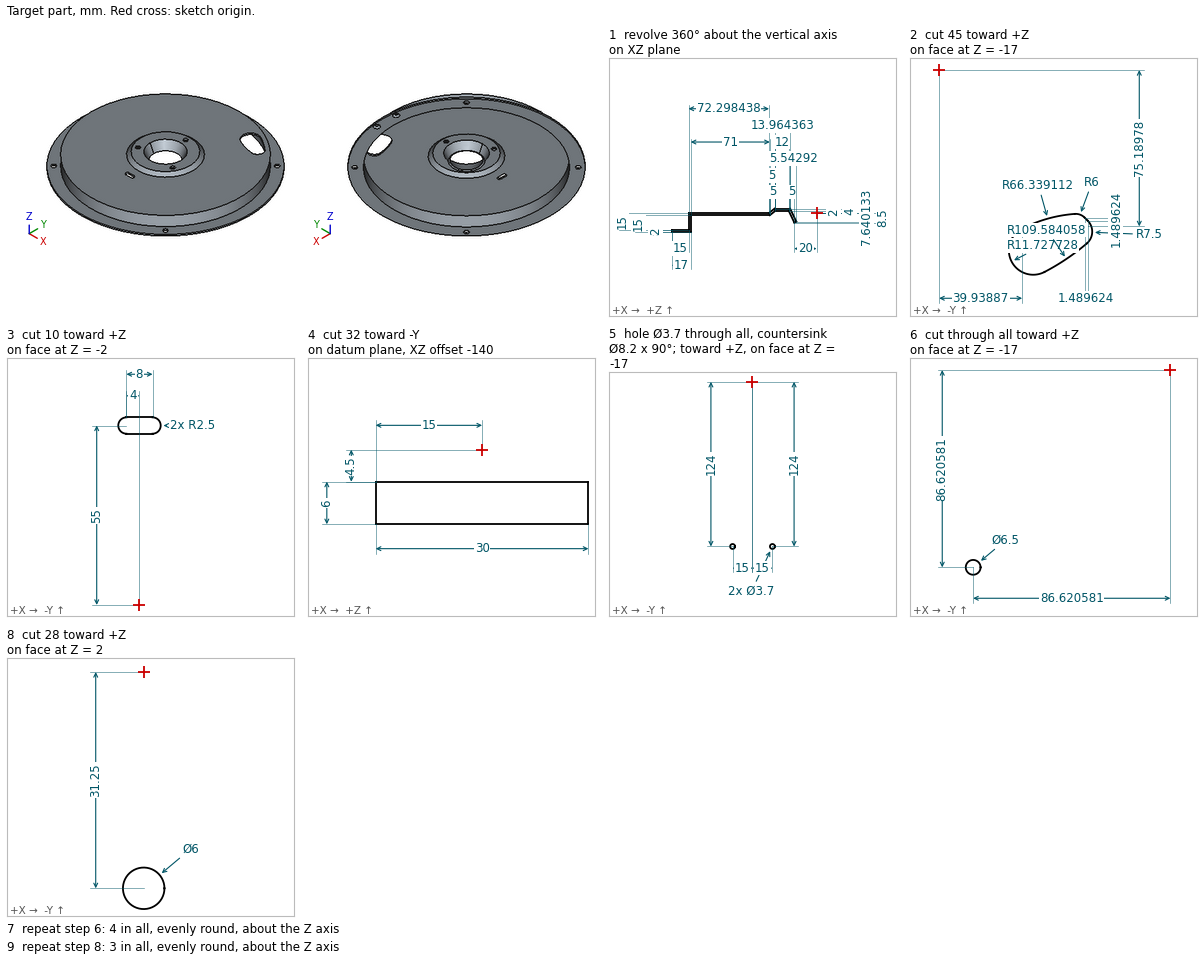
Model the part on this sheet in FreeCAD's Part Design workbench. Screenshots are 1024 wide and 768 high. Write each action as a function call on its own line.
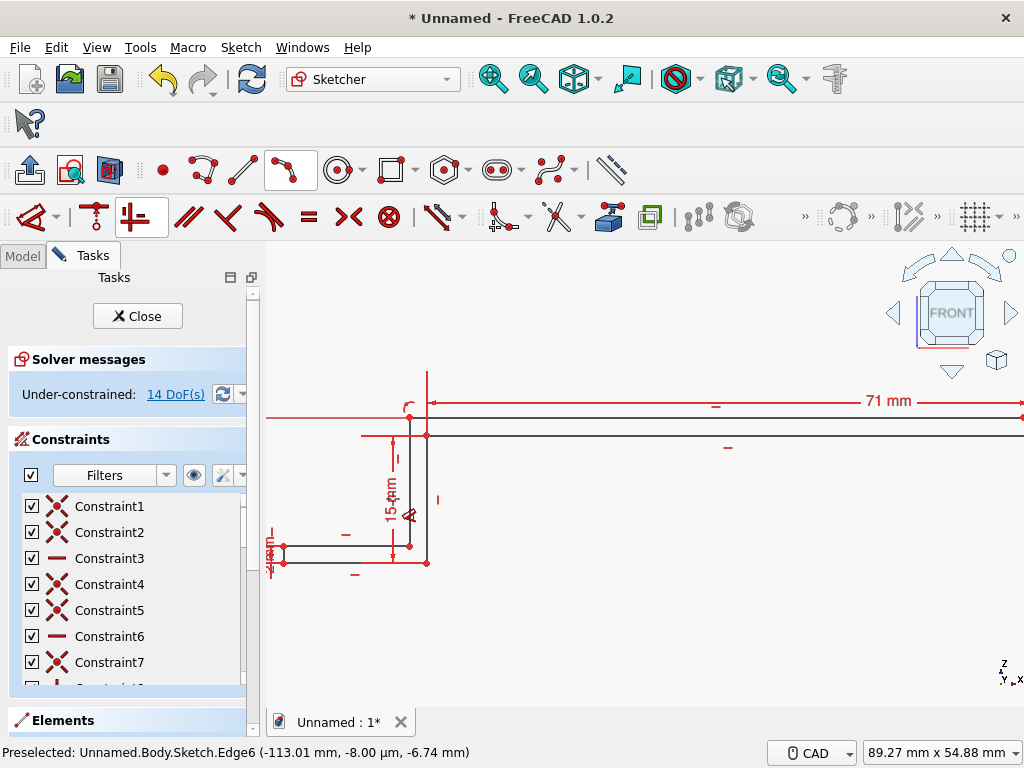
click(384, 563)
click(360, 597)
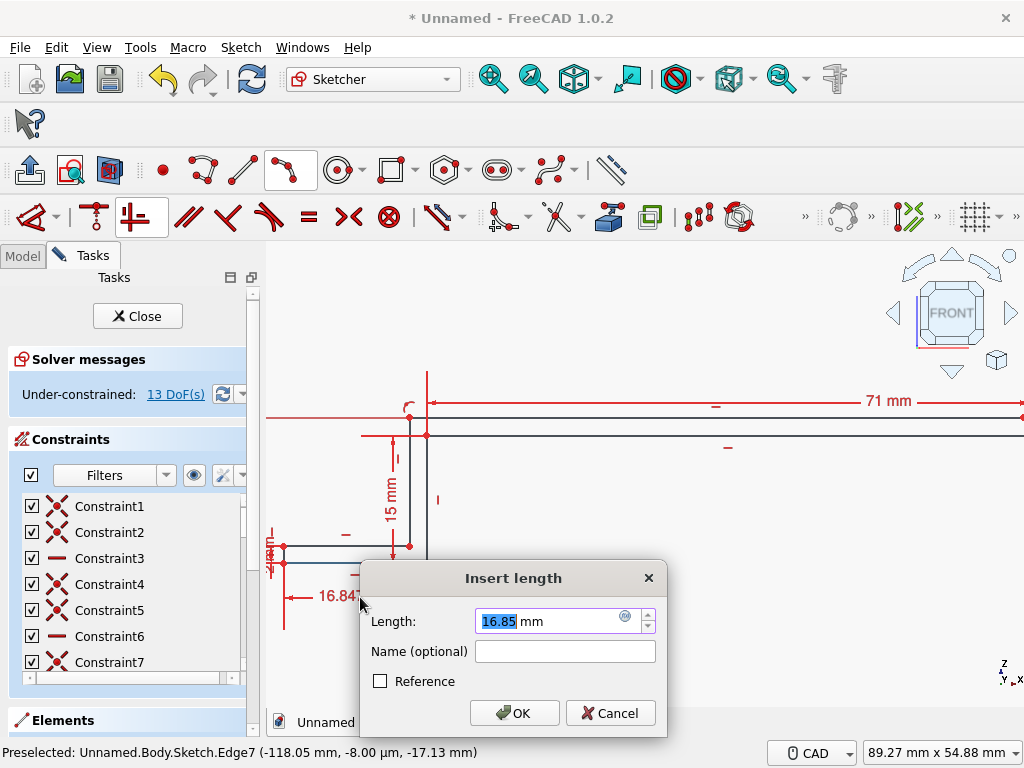
text(17)
key(Return)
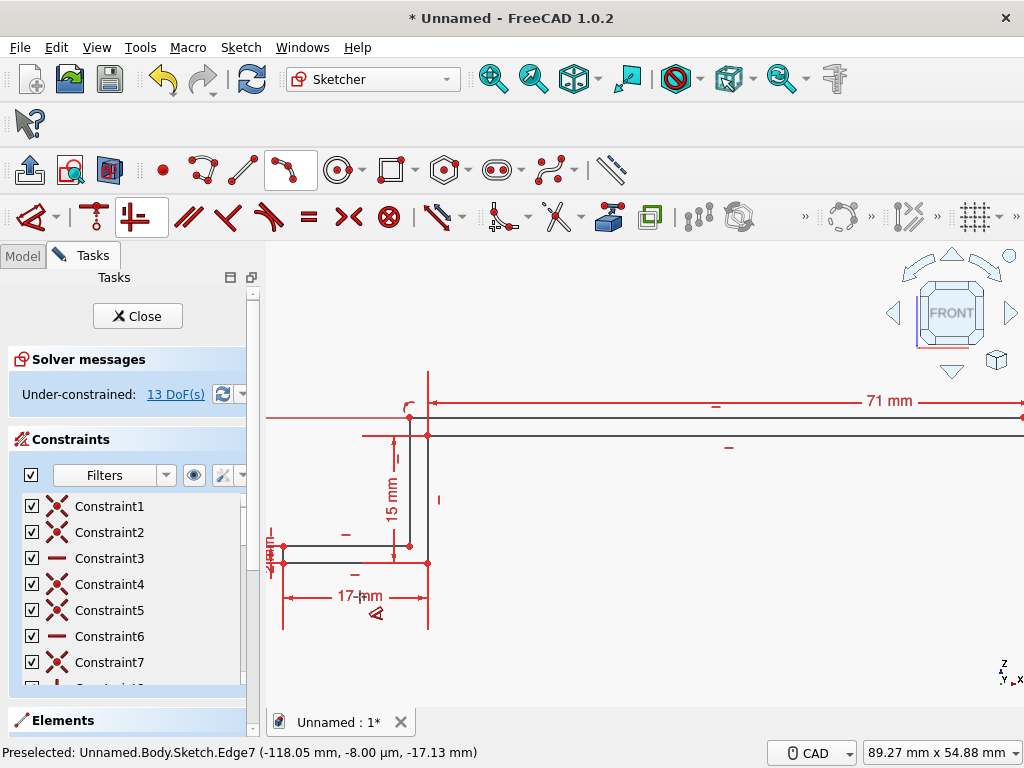
click(321, 546)
click(311, 512)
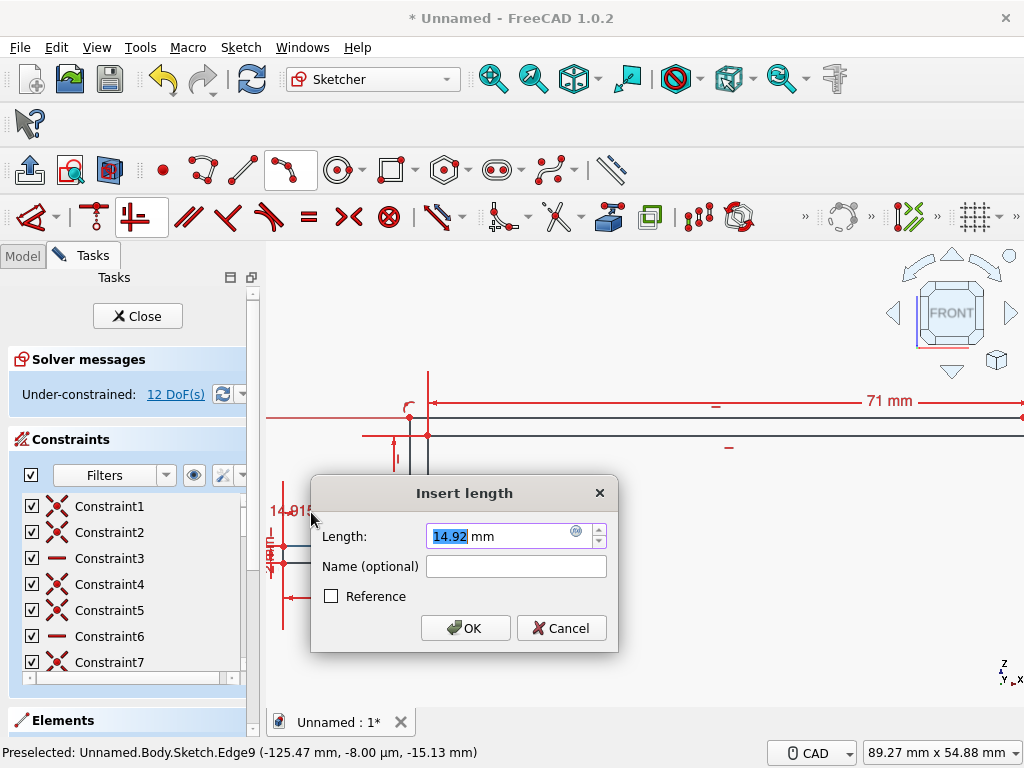
text(15)
key(Return)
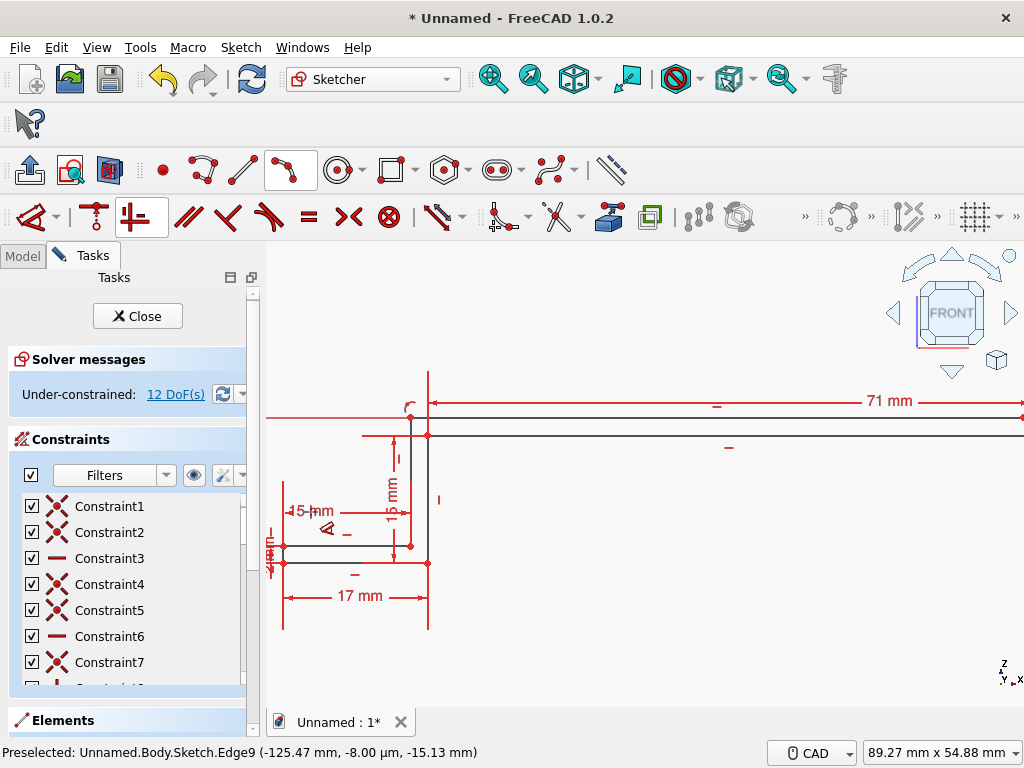
click(411, 508)
click(377, 452)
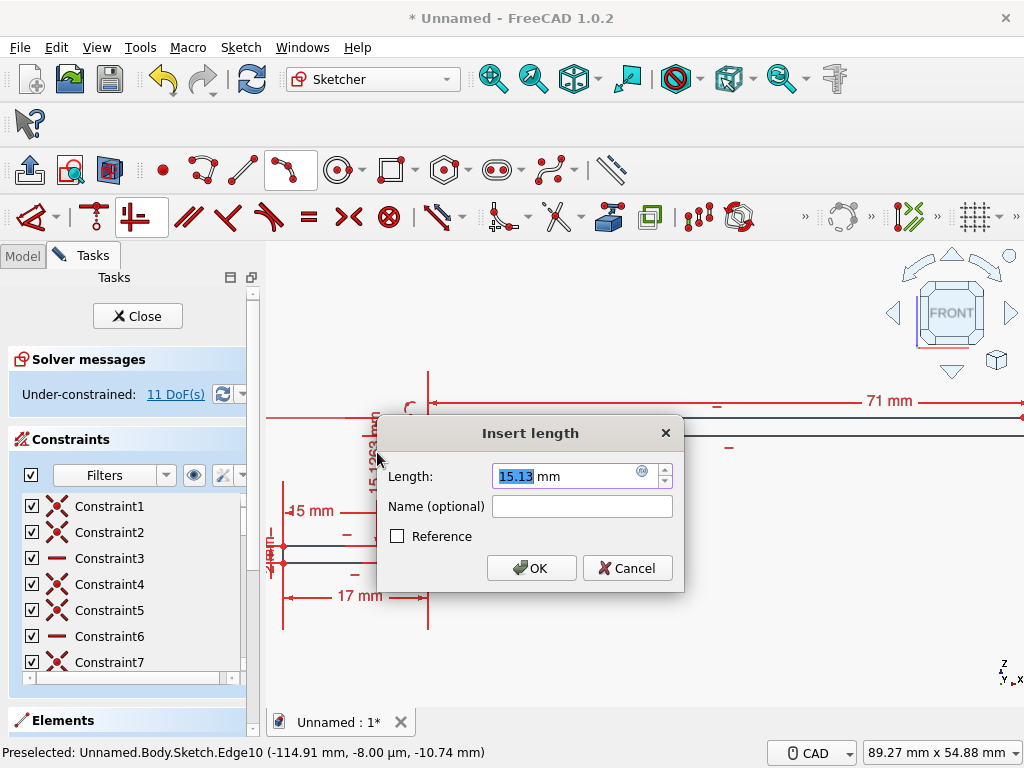
text(15)
key(Return)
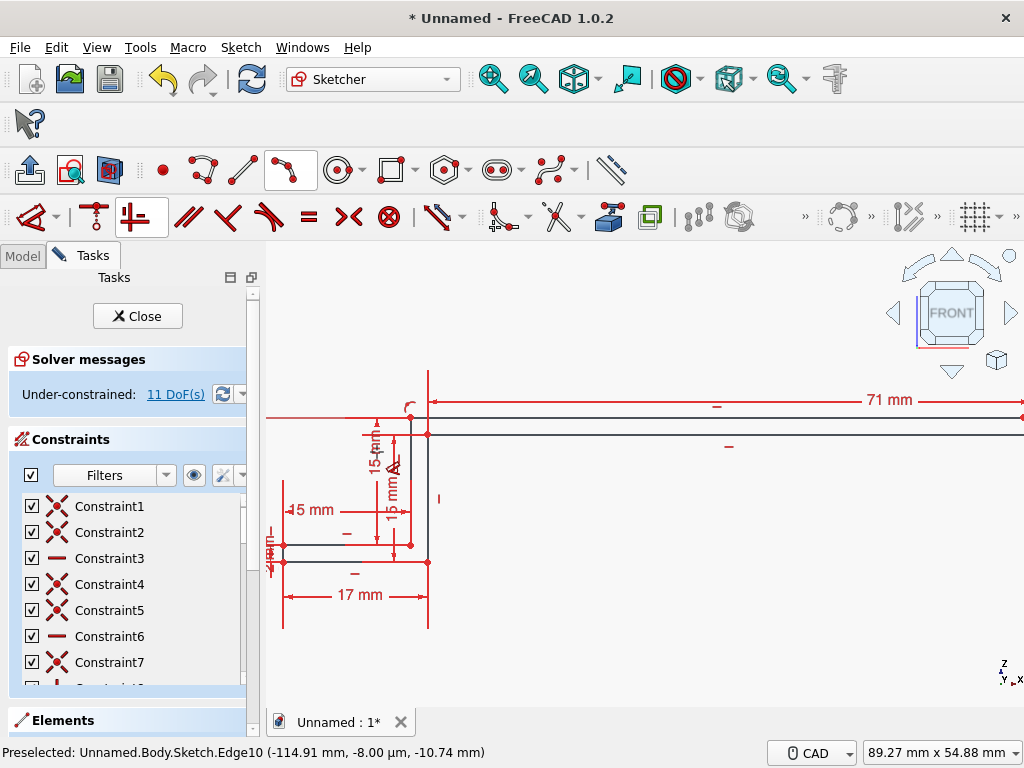
scroll(426, 475, down, 5)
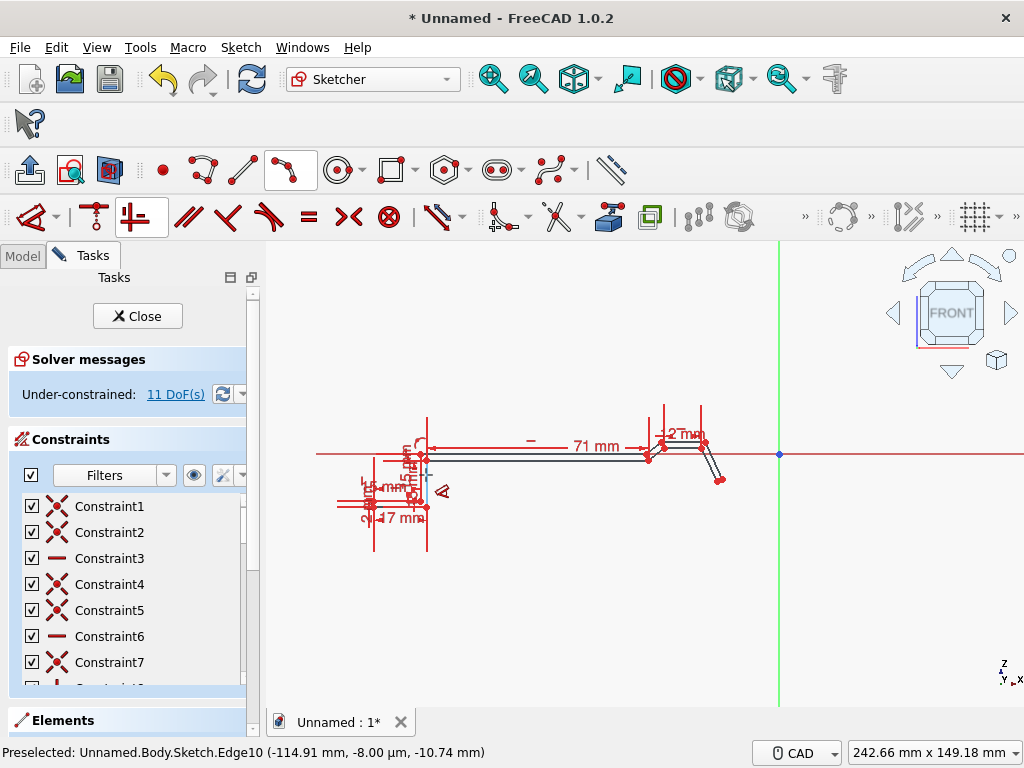
scroll(701, 448, up, 10)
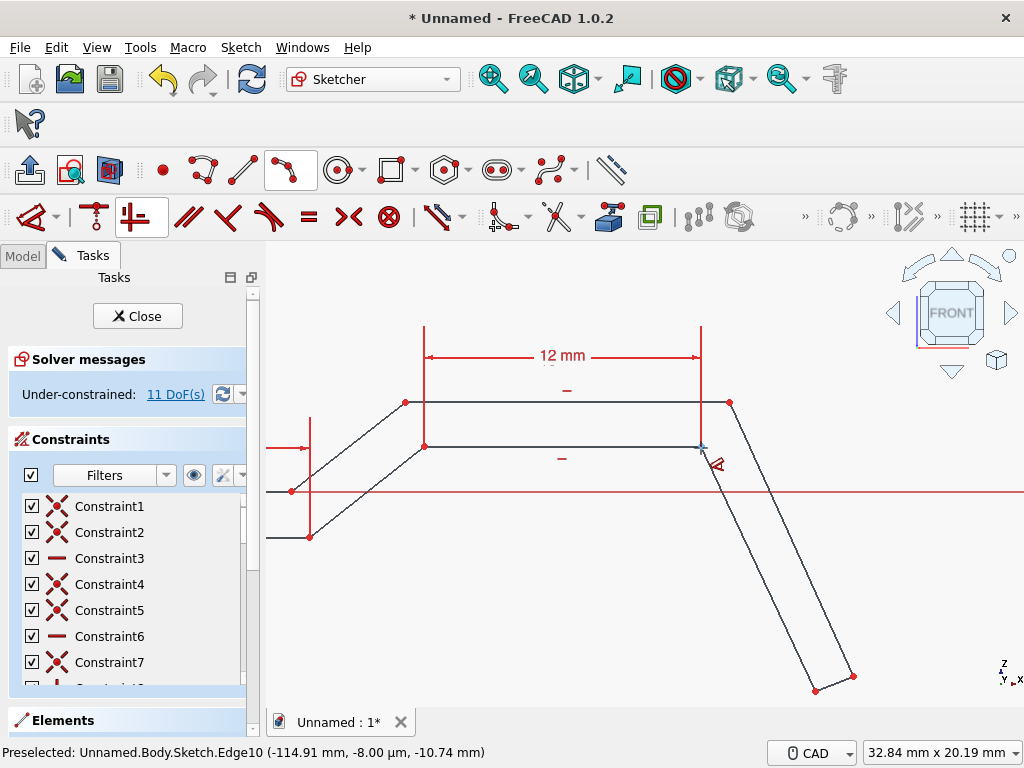
click(701, 447)
click(667, 469)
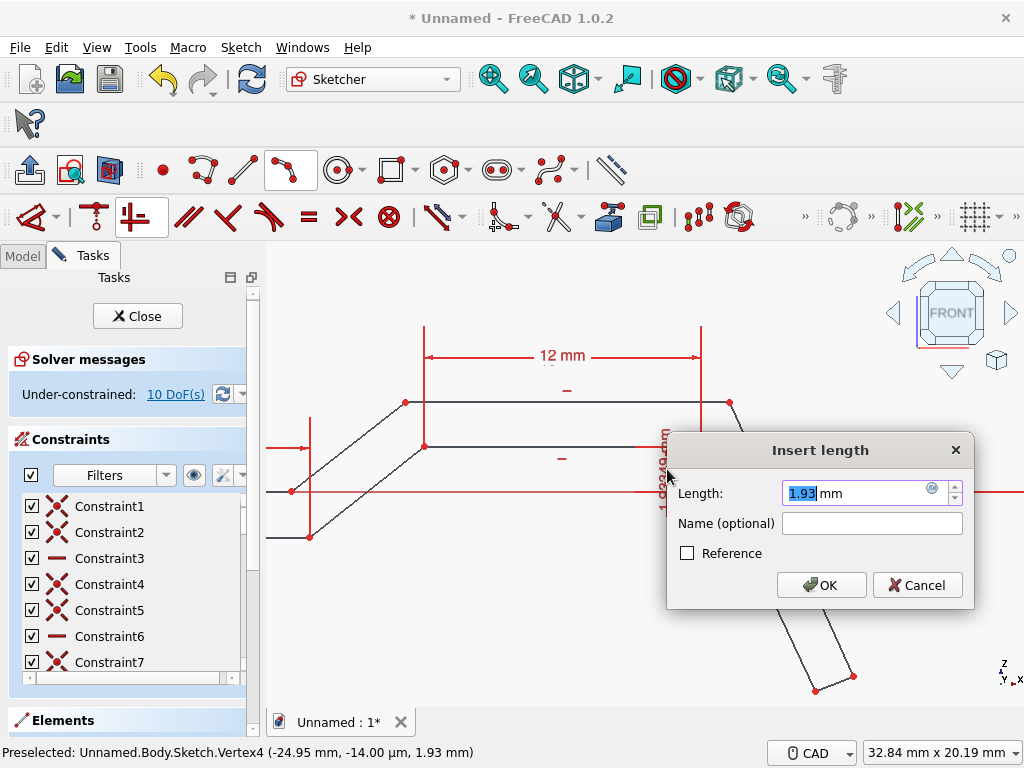
text(2)
key(Return)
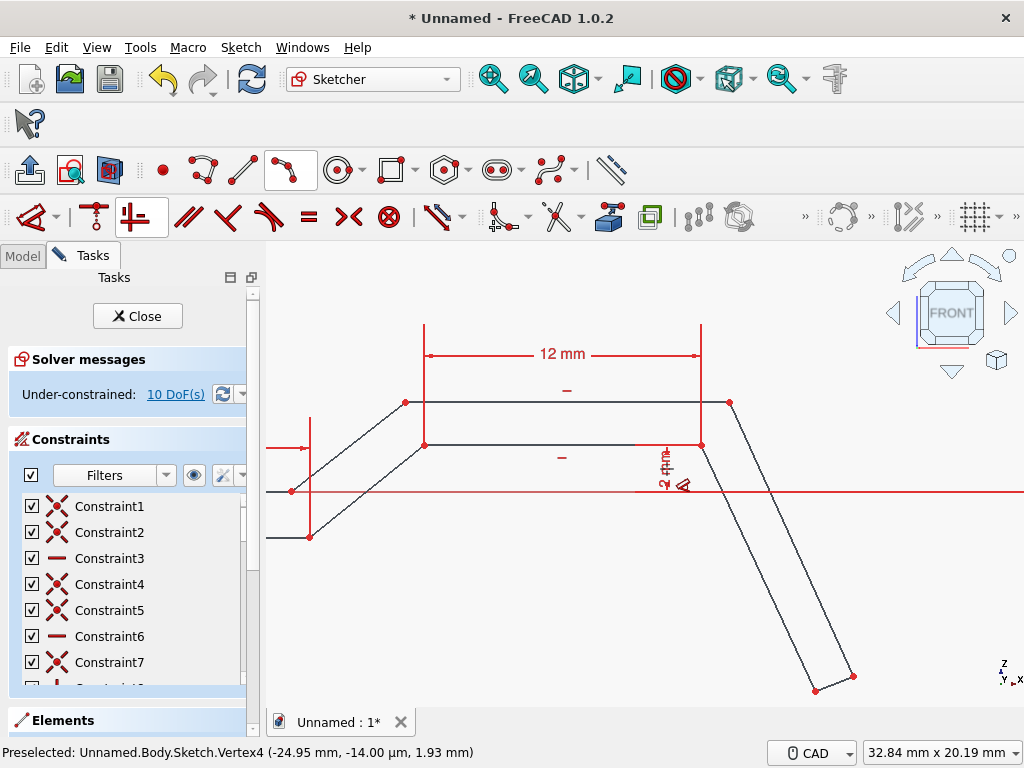
click(406, 402)
click(372, 447)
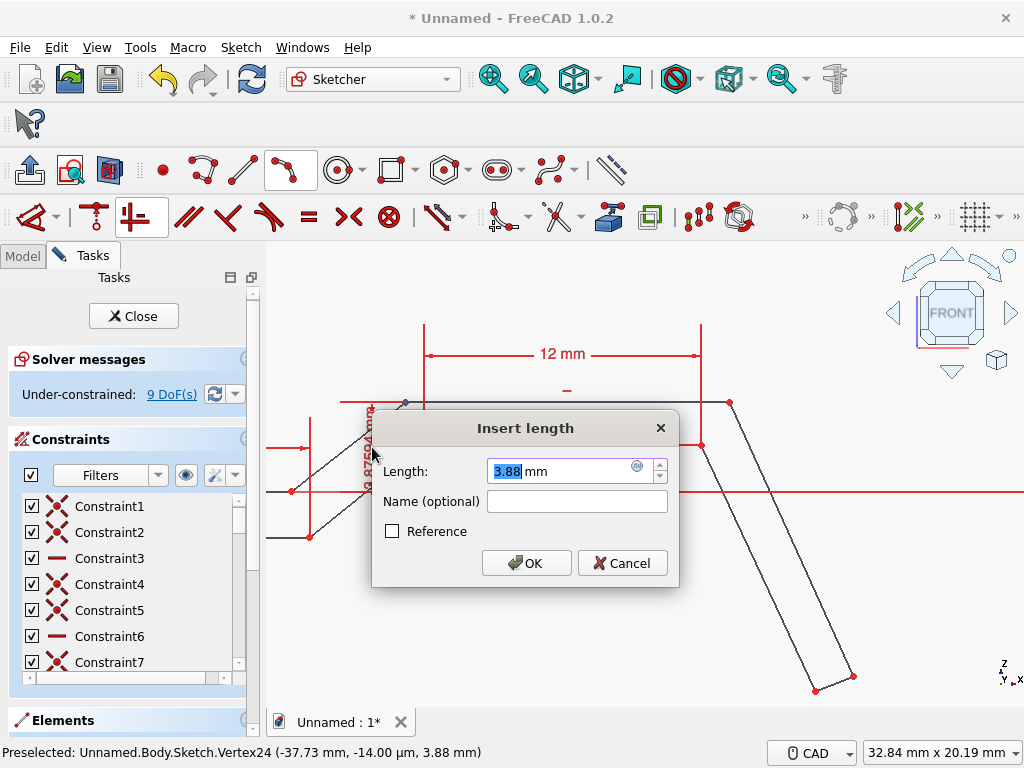
text(4)
key(Return)